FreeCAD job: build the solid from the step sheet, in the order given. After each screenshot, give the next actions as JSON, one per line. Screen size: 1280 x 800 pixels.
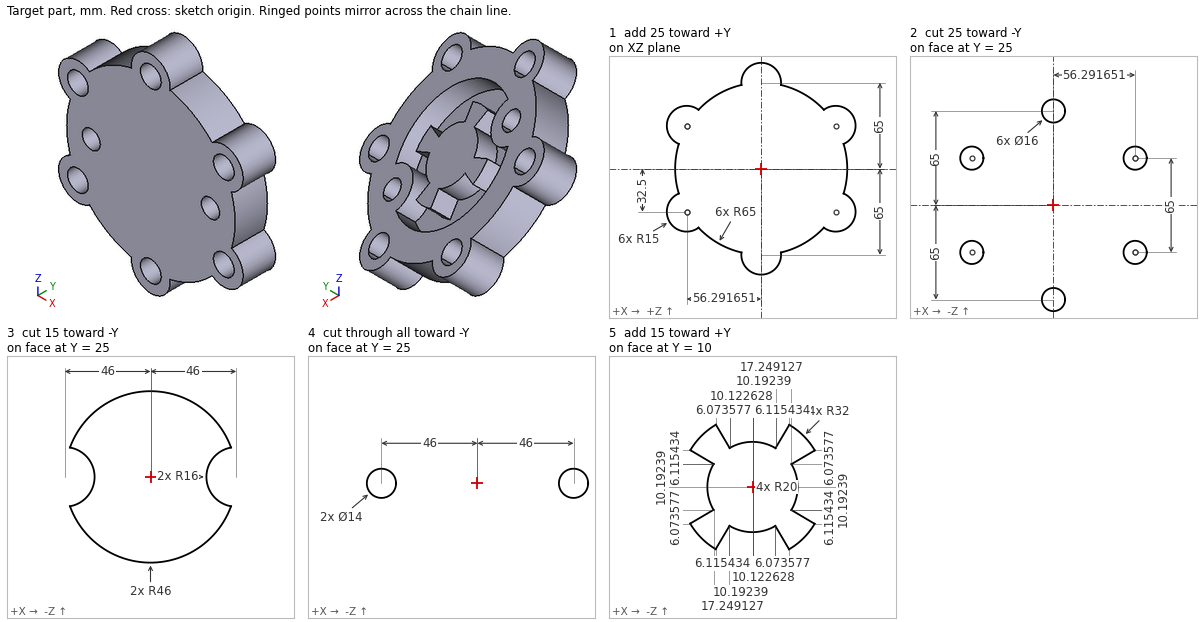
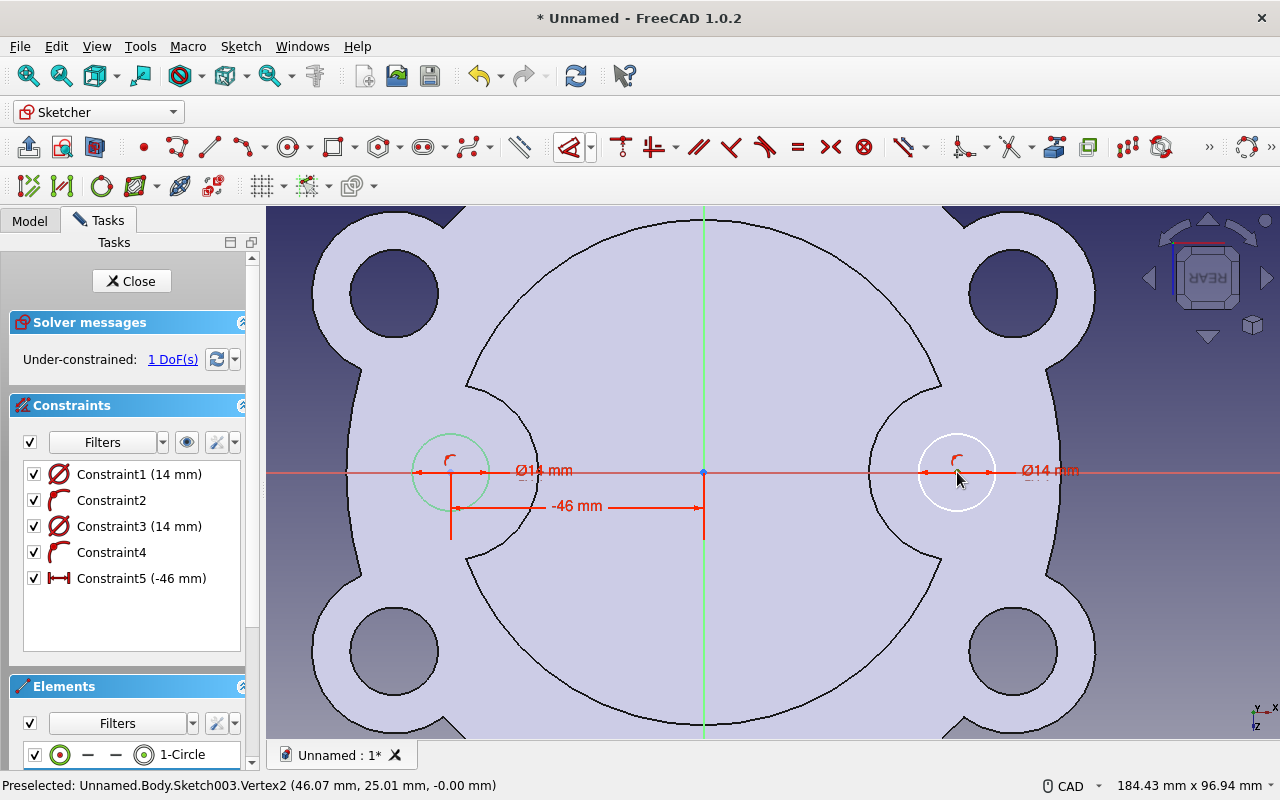
{"action": "key", "text": "l"}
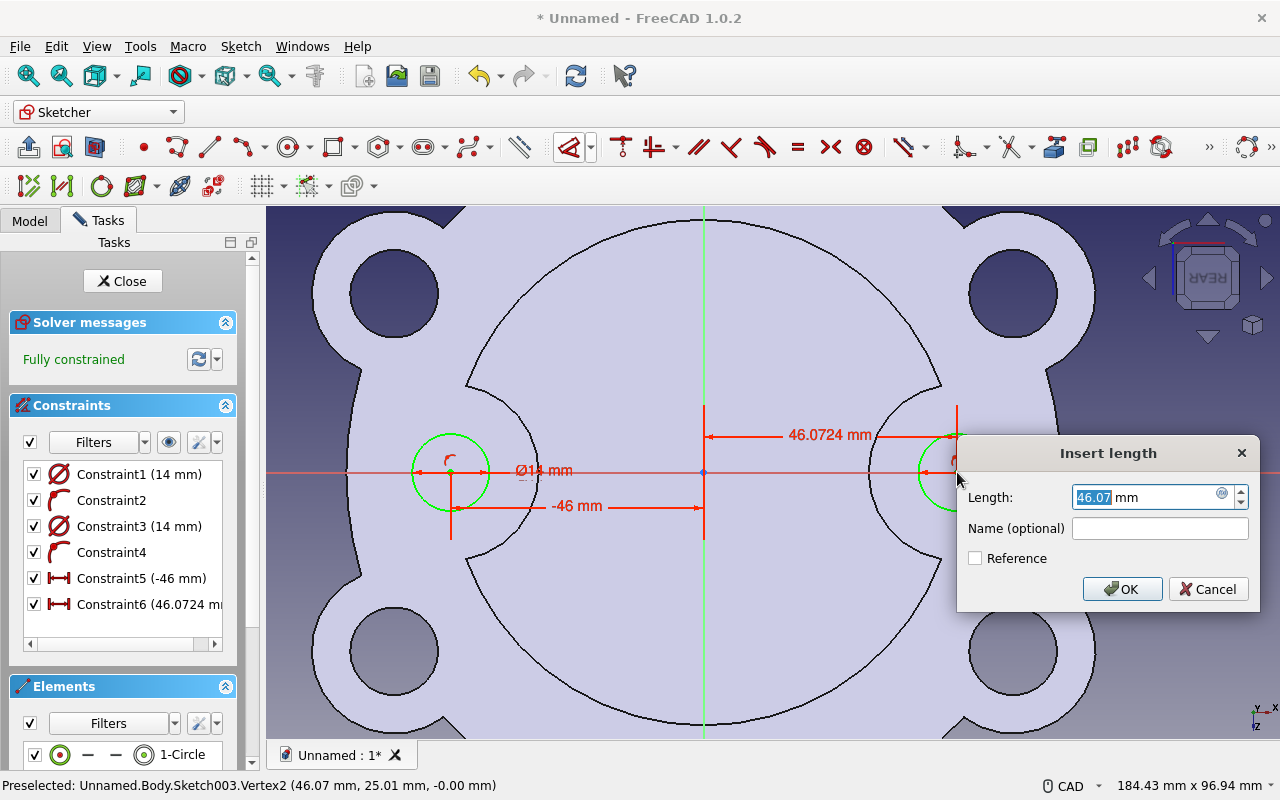
{"action": "type", "text": "46"}
{"action": "key", "text": "Return"}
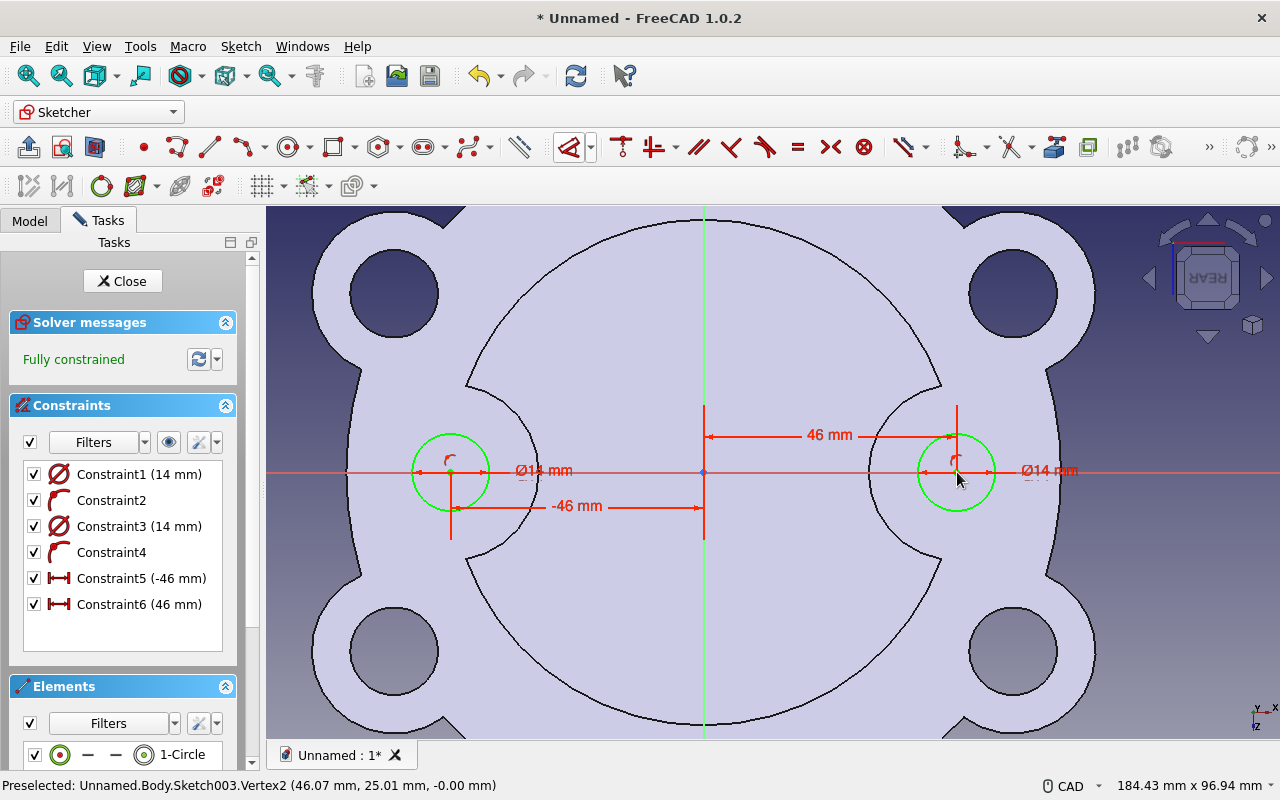
{"action": "left_click", "coordinate": [123, 281]}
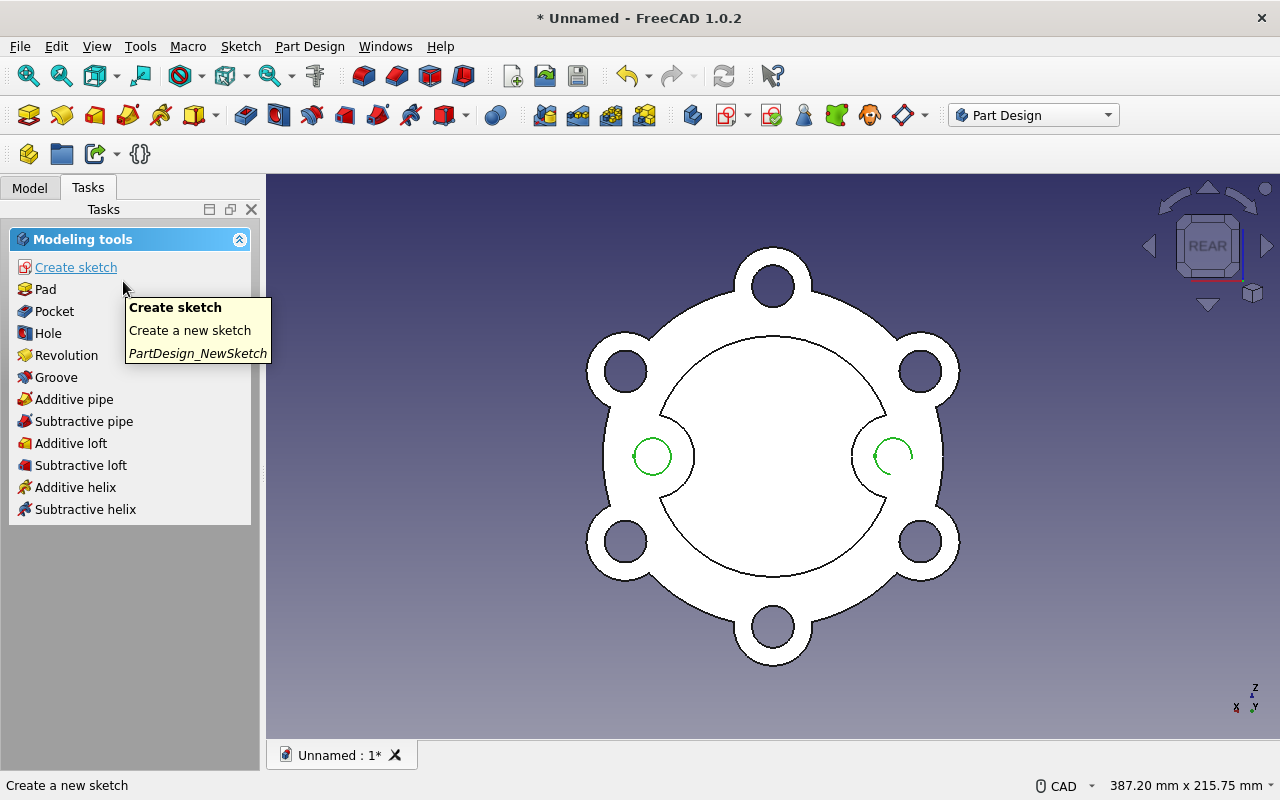
{"action": "left_click", "coordinate": [246, 116]}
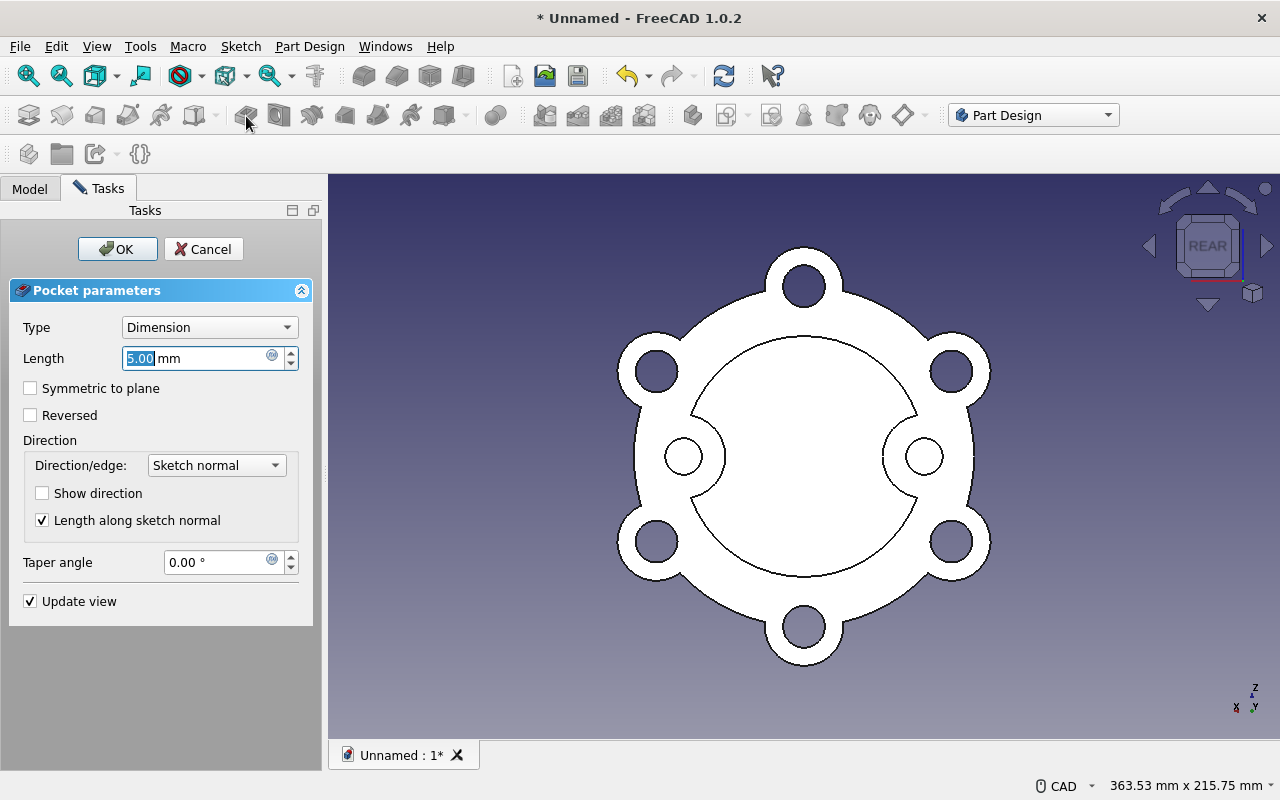
{"action": "left_click", "coordinate": [210, 328]}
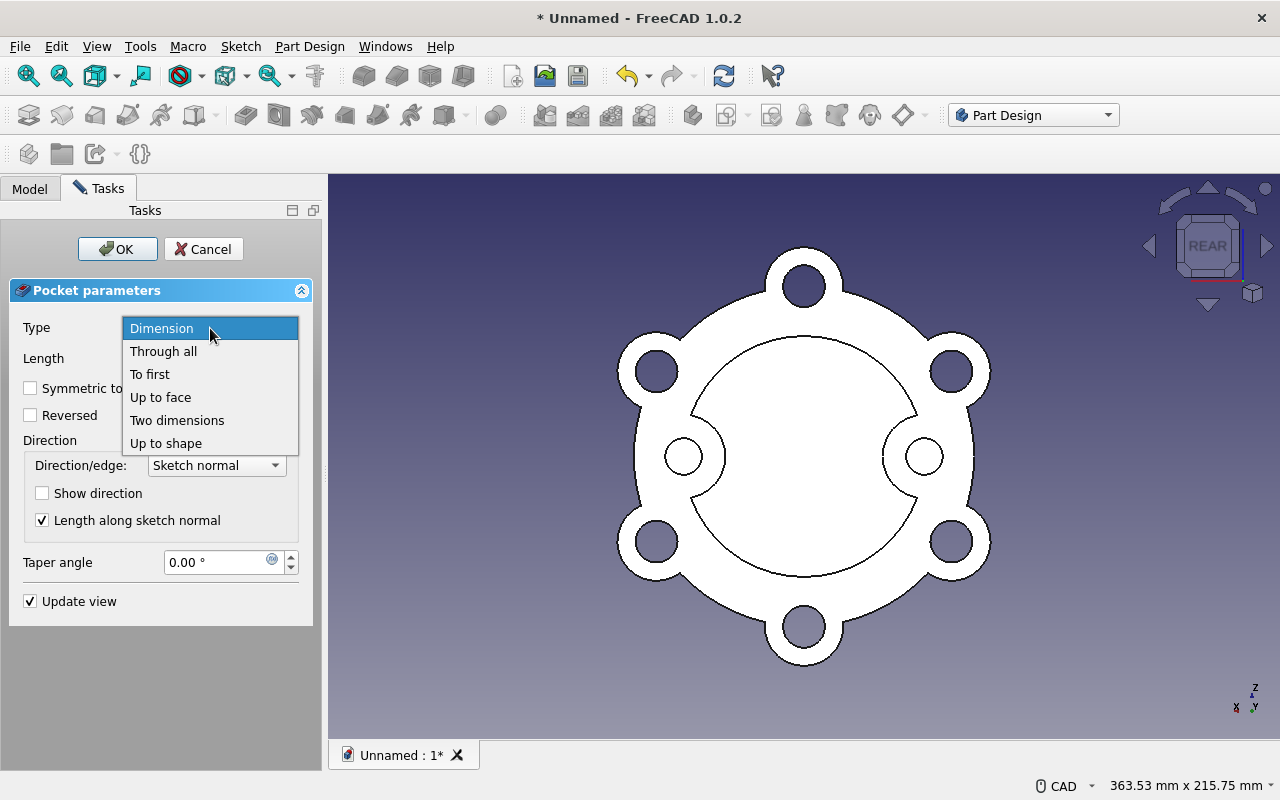
{"action": "left_click", "coordinate": [208, 352]}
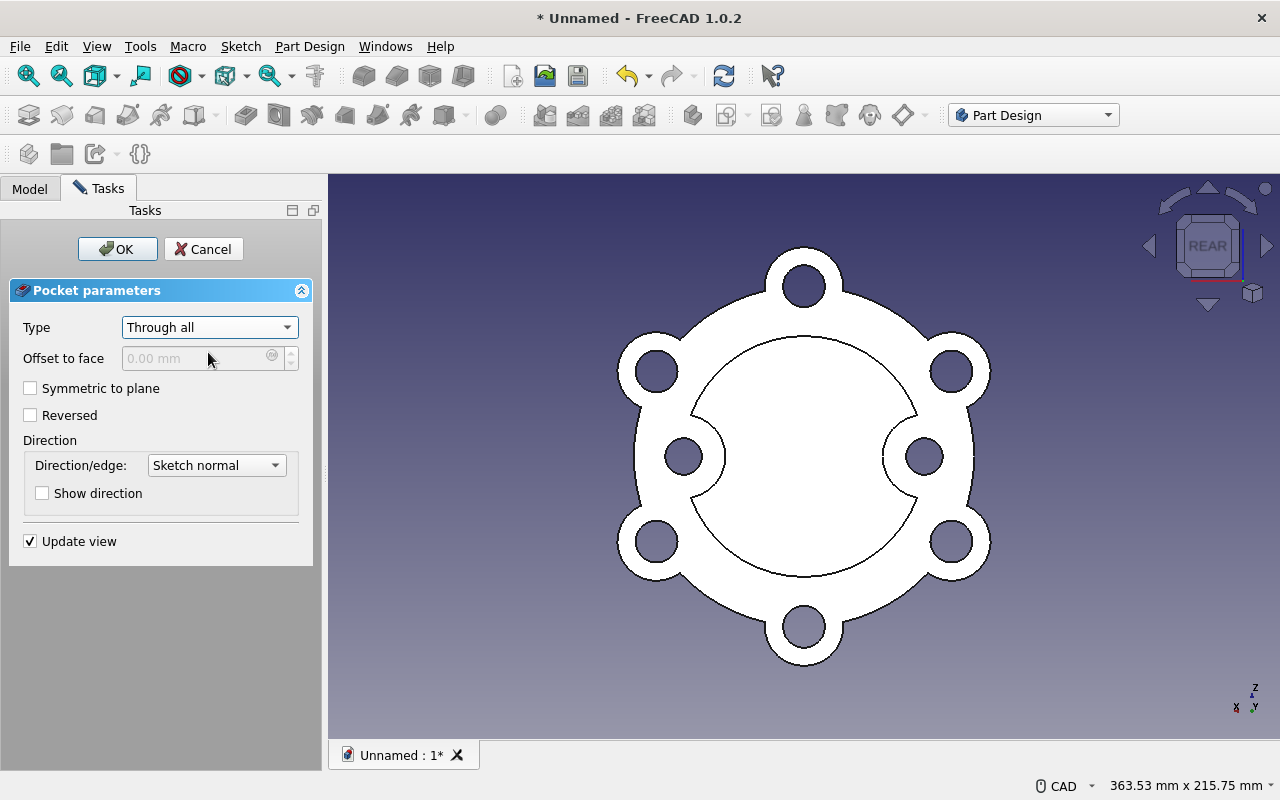
{"action": "left_click", "coordinate": [118, 249]}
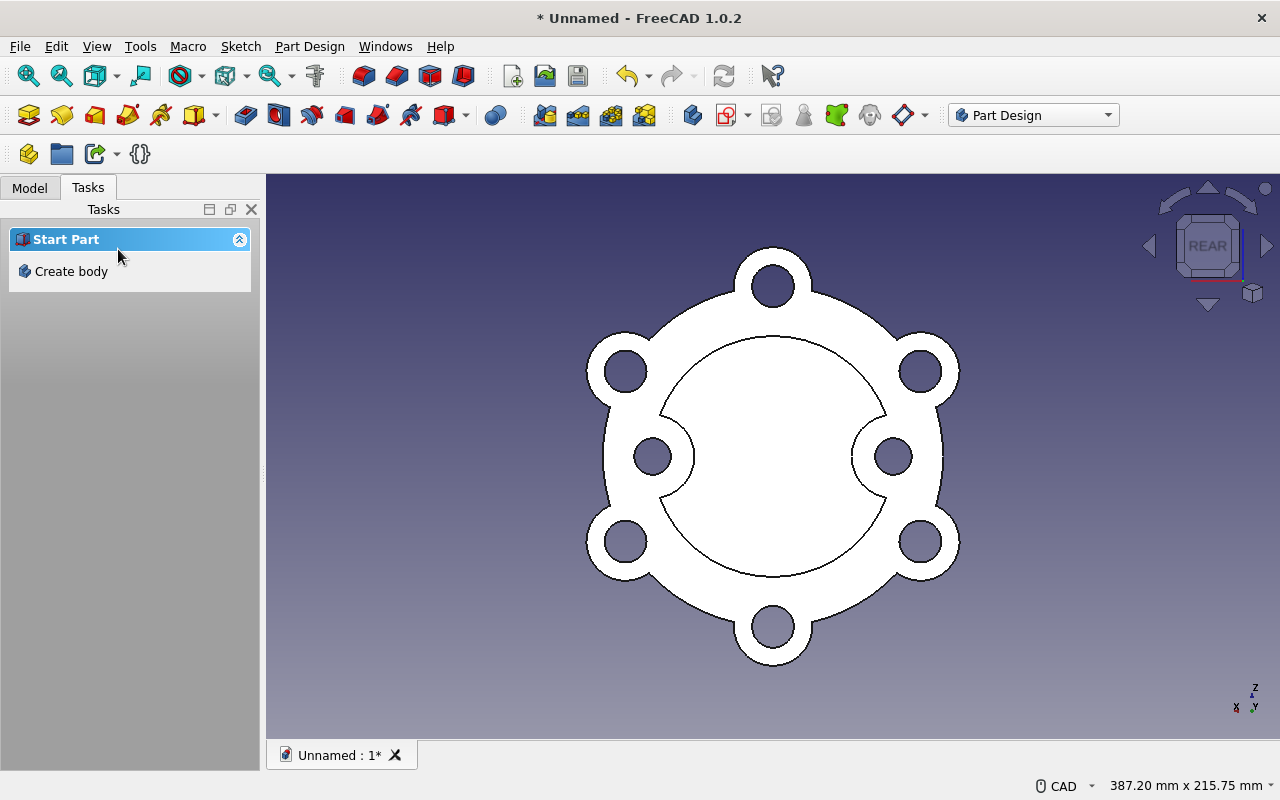
{"action": "left_click", "coordinate": [773, 490]}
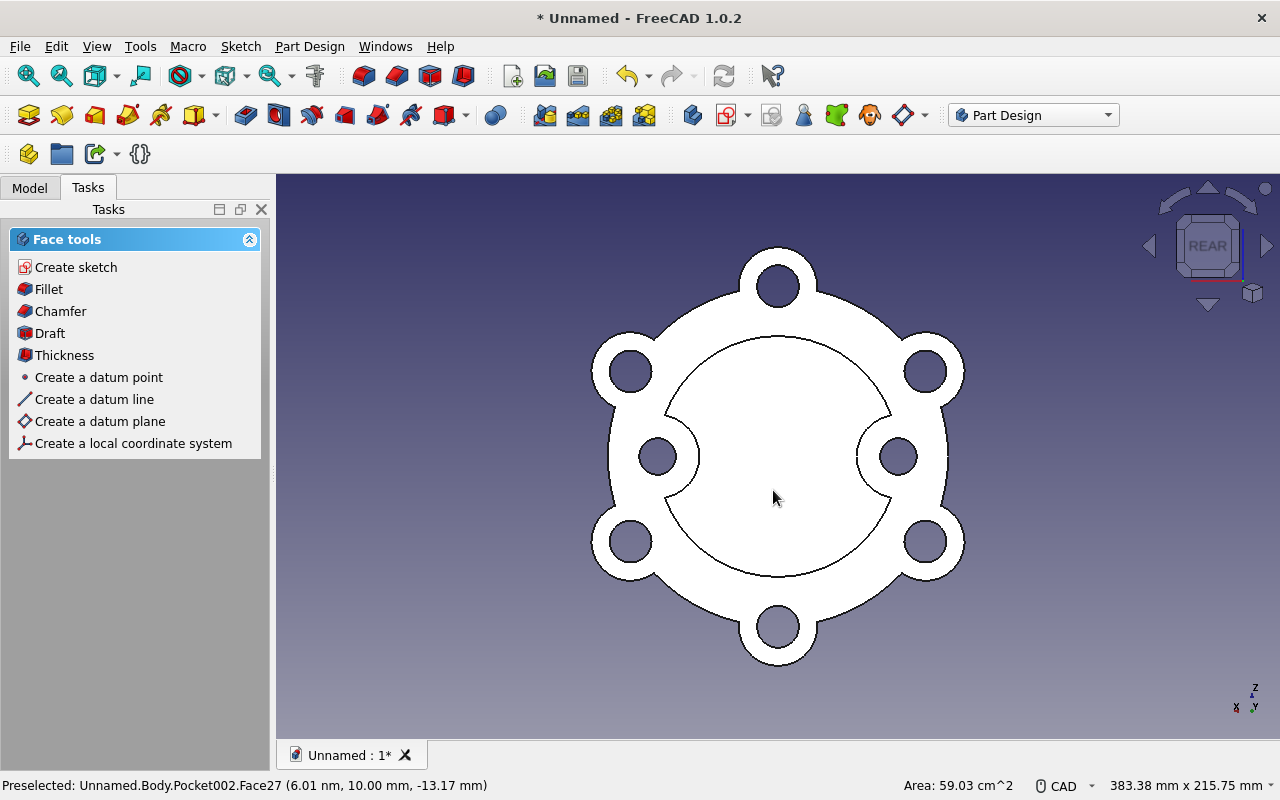
{"action": "left_click", "coordinate": [726, 116]}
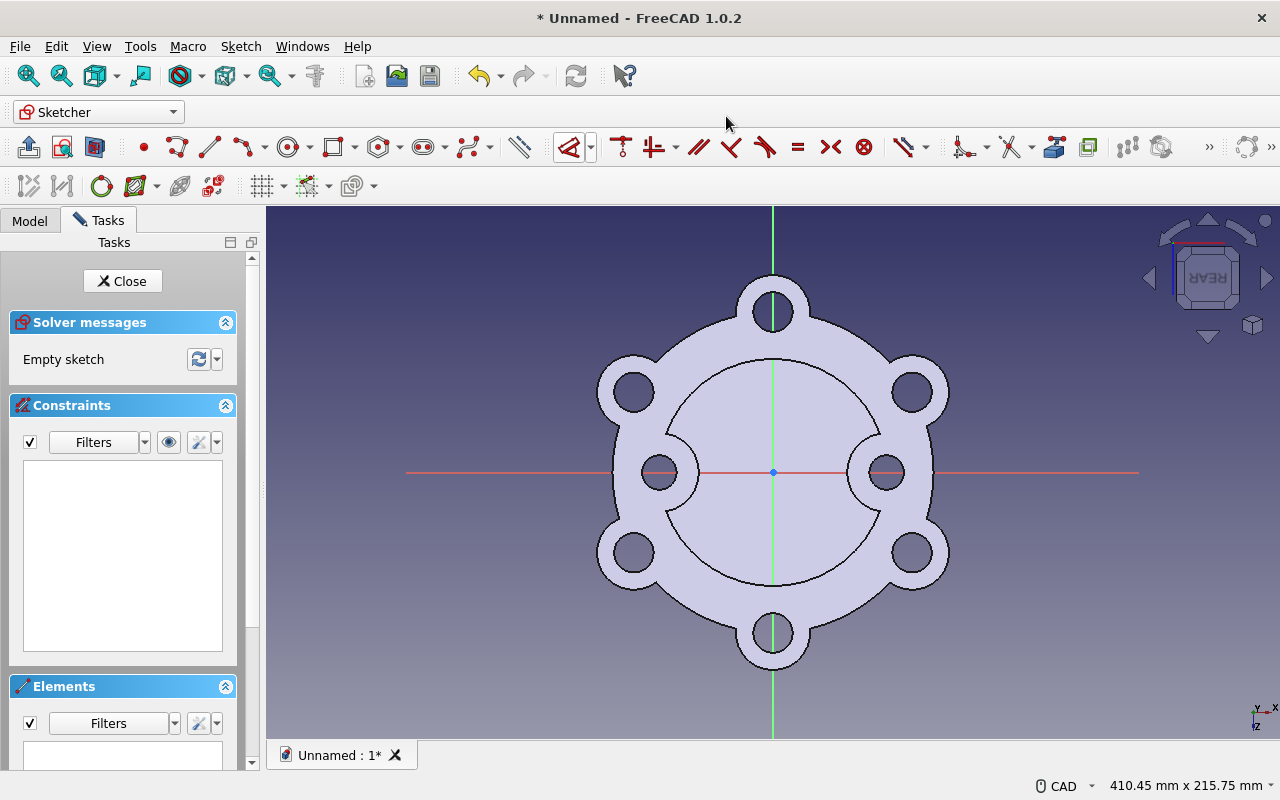
{"action": "left_click", "coordinate": [95, 148]}